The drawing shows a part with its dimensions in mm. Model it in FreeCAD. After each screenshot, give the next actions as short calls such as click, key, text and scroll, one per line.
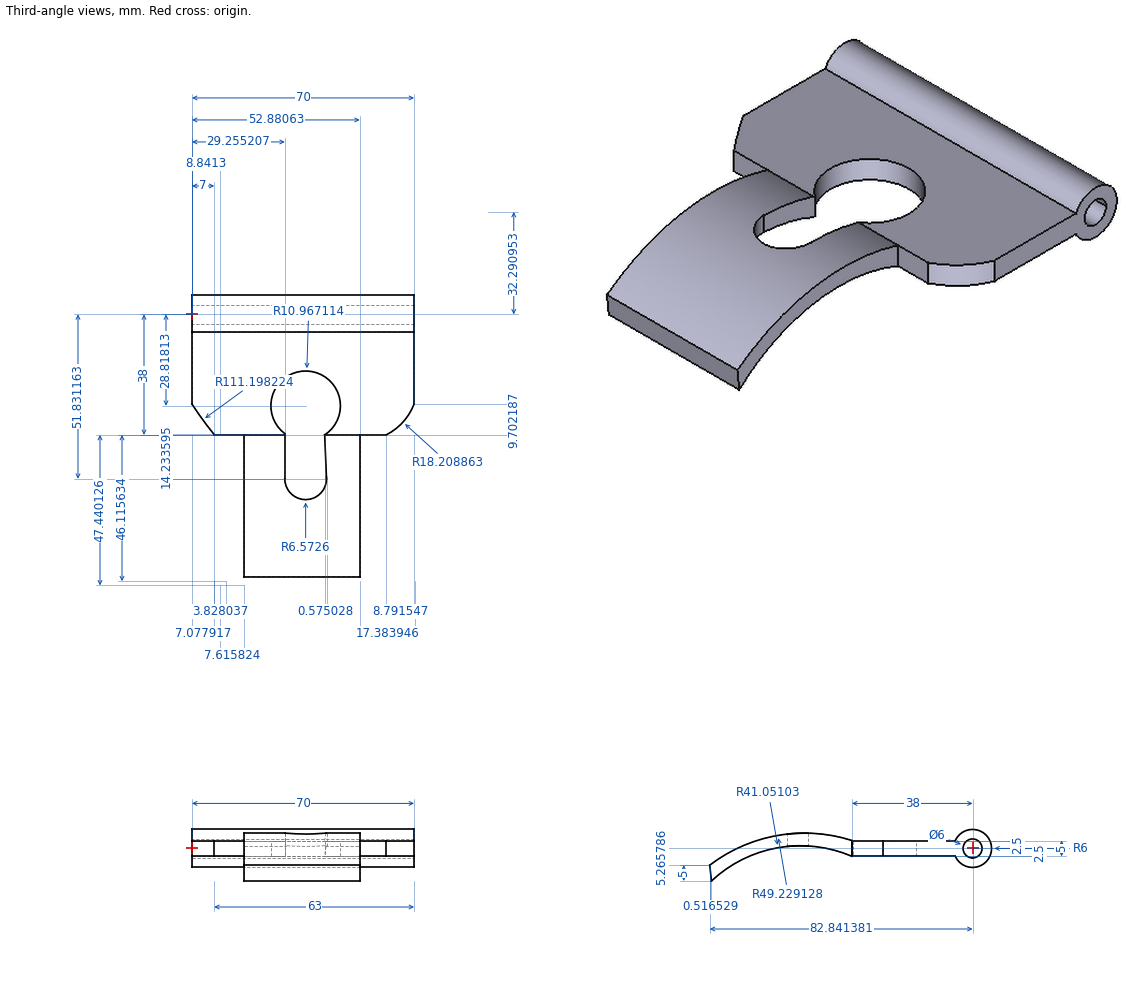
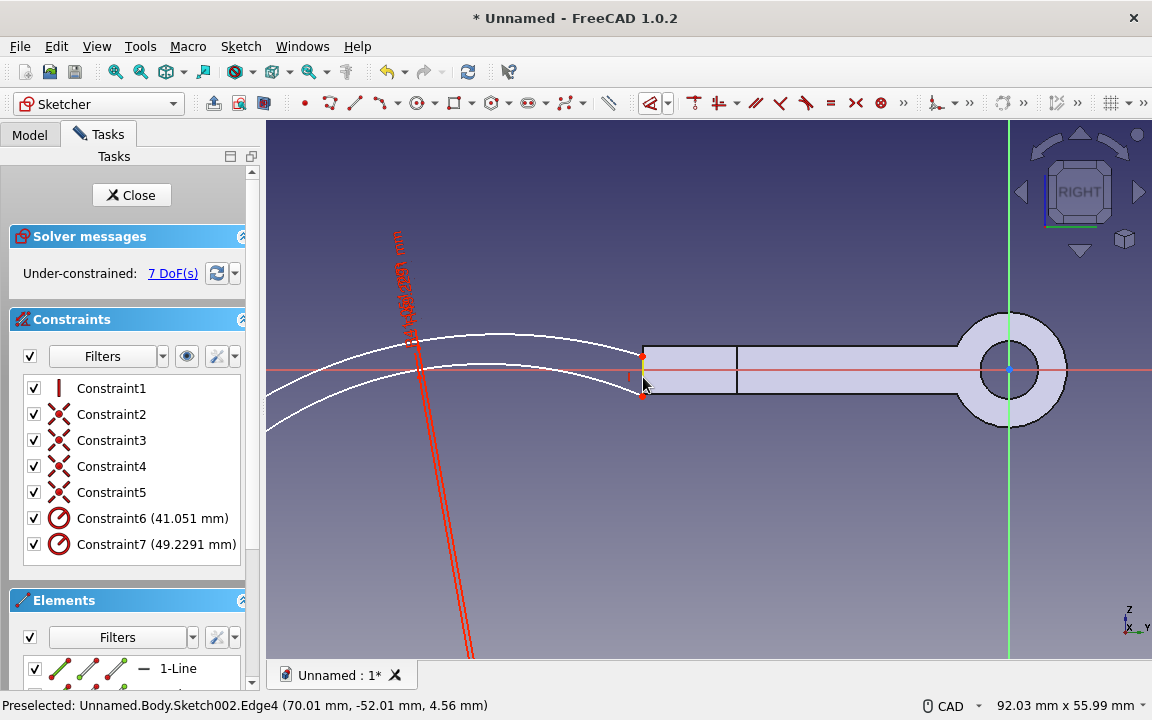
click(643, 376)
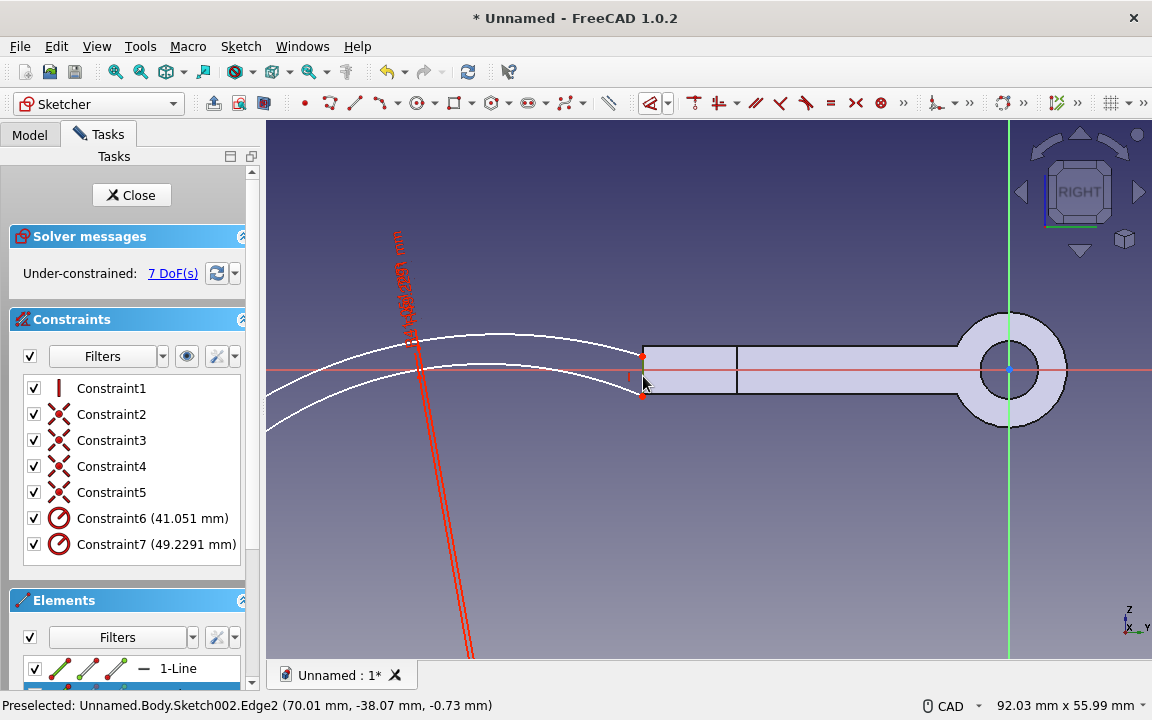
key(i)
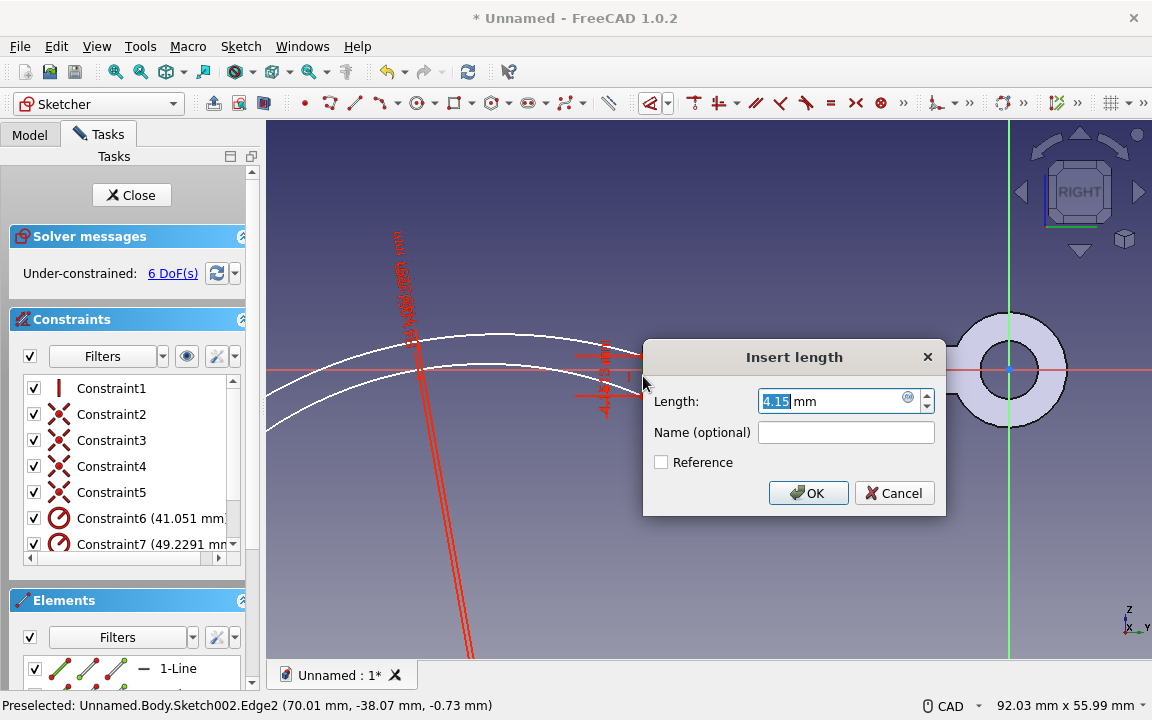
text(5)
key(Return)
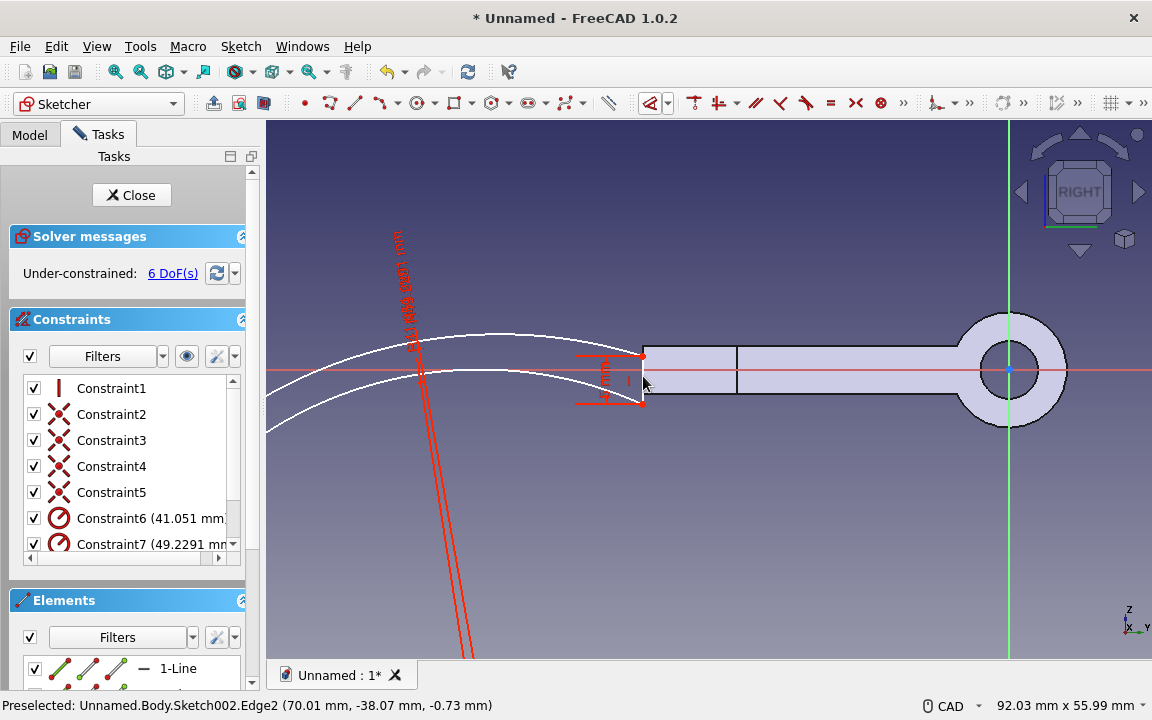
scroll(702, 369, down, 2)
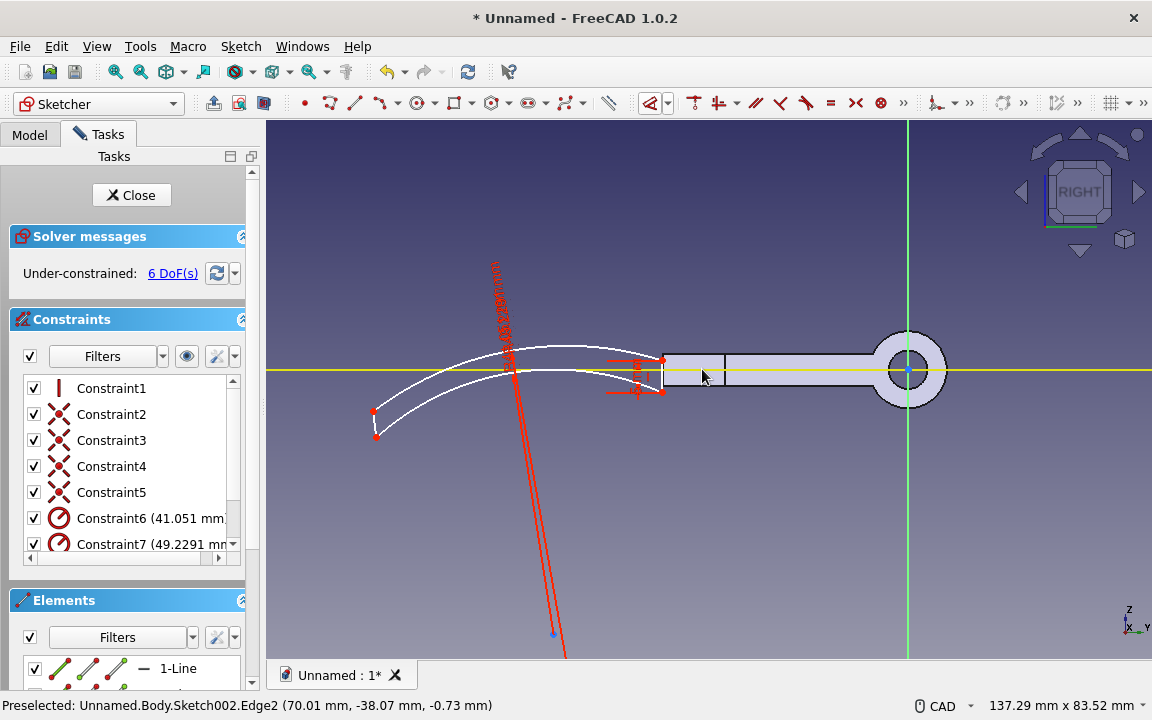
scroll(374, 419, up, 3)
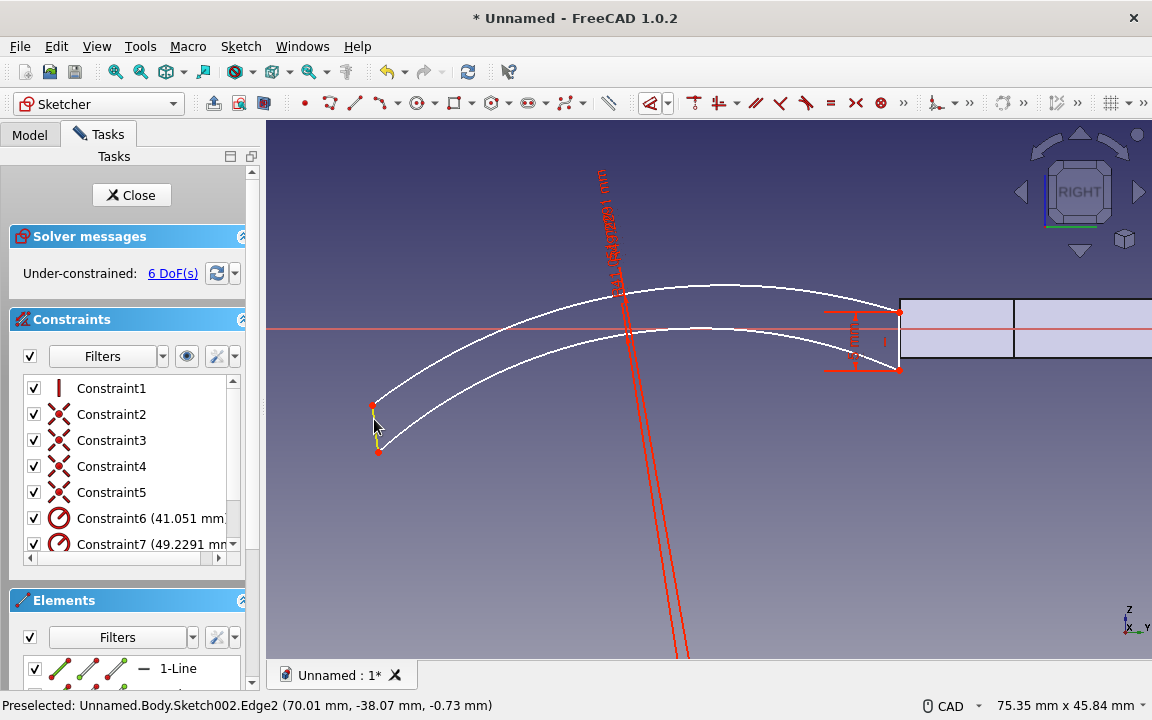
click(374, 419)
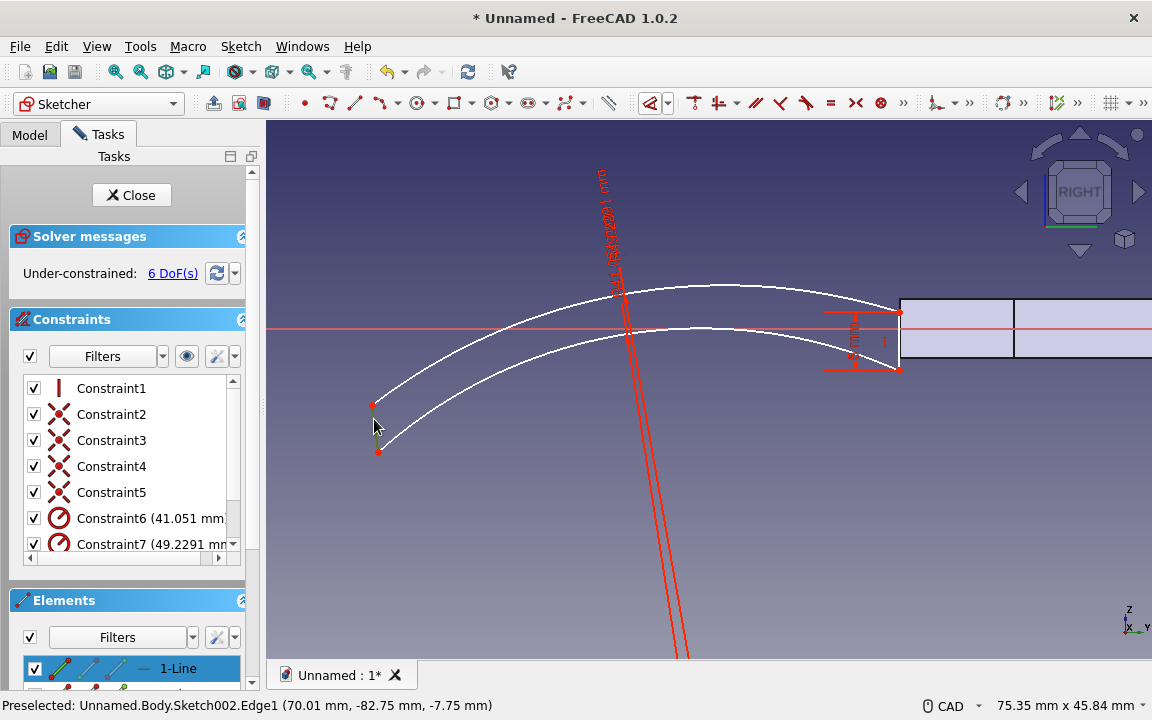
click(668, 104)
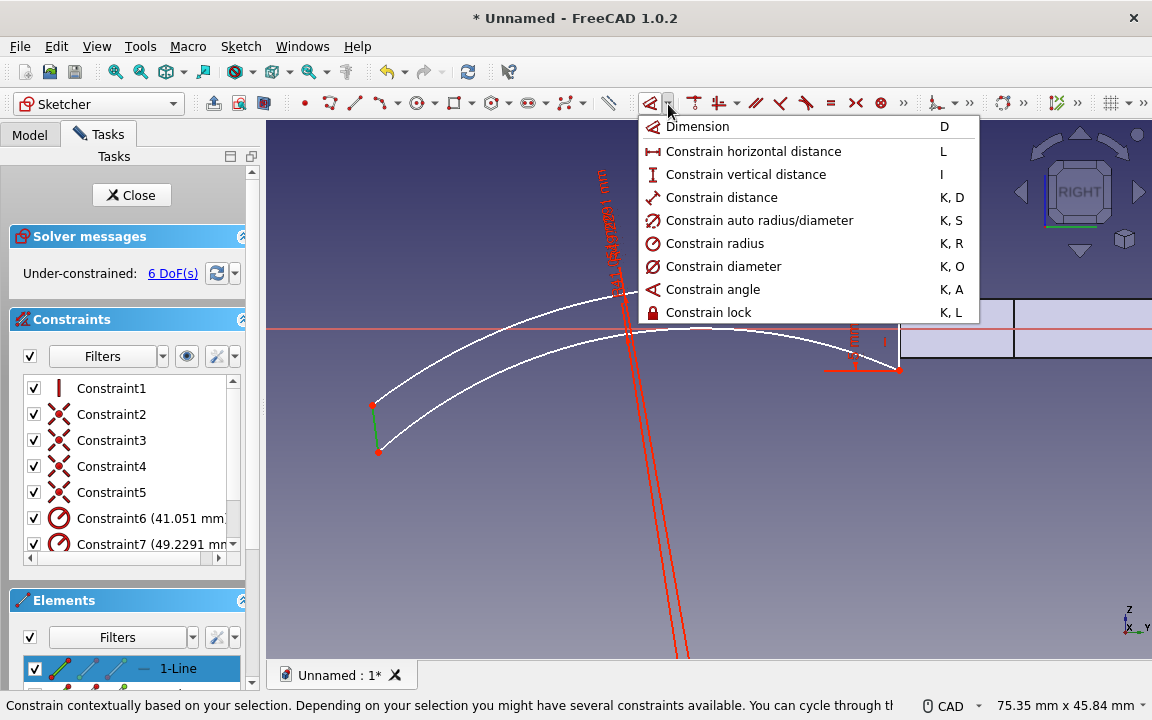
click(809, 174)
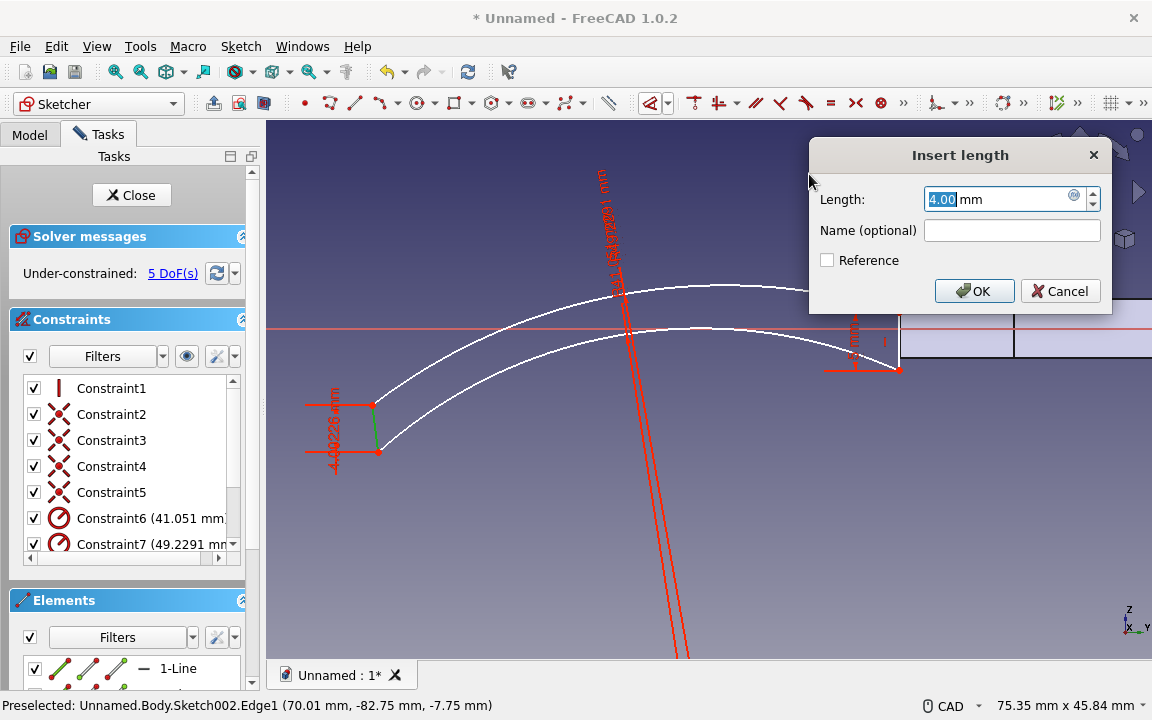
text(5)
key(Return)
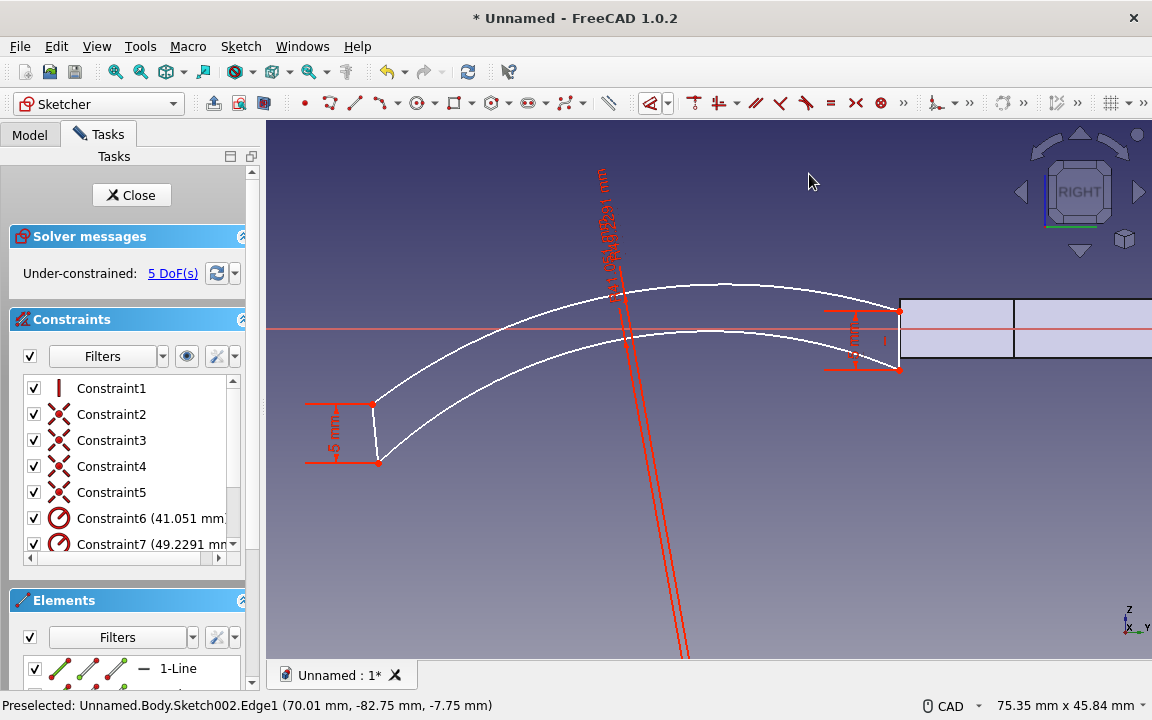
click(899, 370)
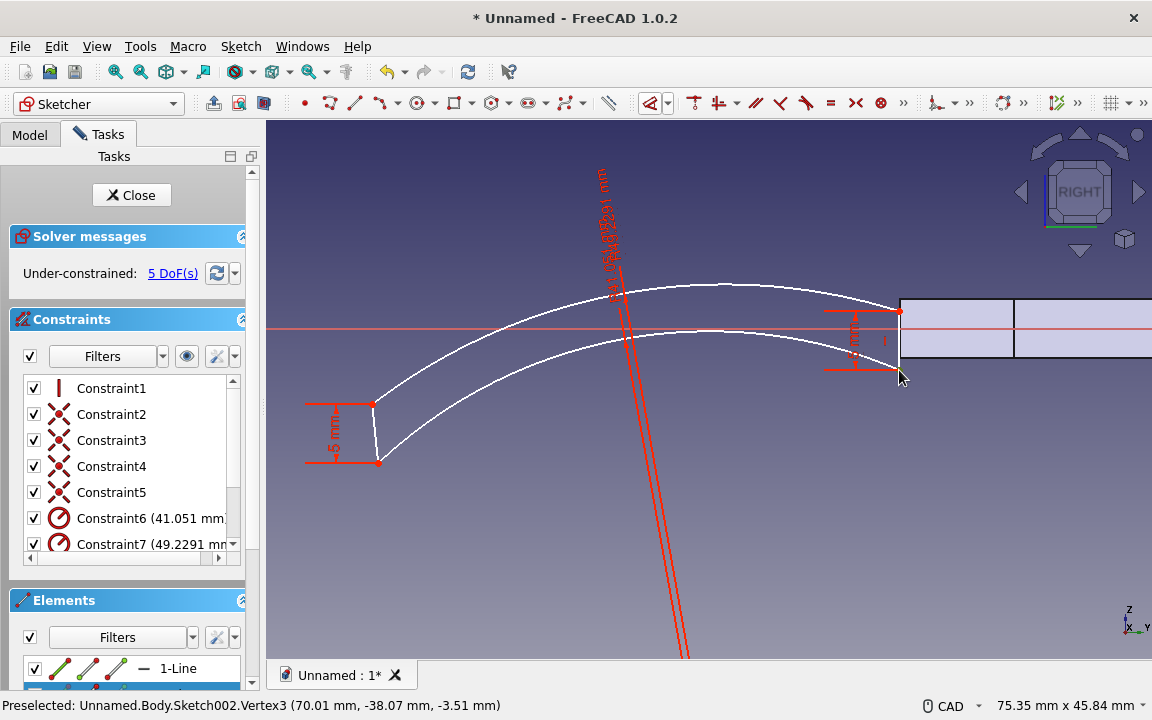
key(l)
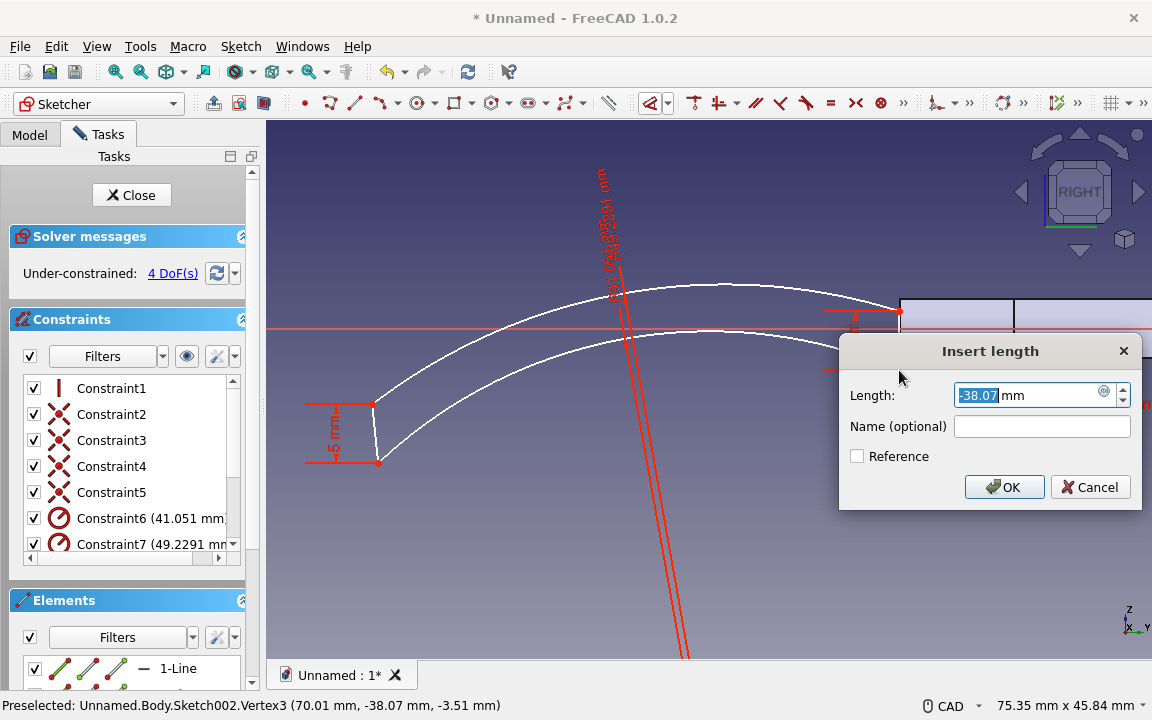
text(-38)
key(Return)